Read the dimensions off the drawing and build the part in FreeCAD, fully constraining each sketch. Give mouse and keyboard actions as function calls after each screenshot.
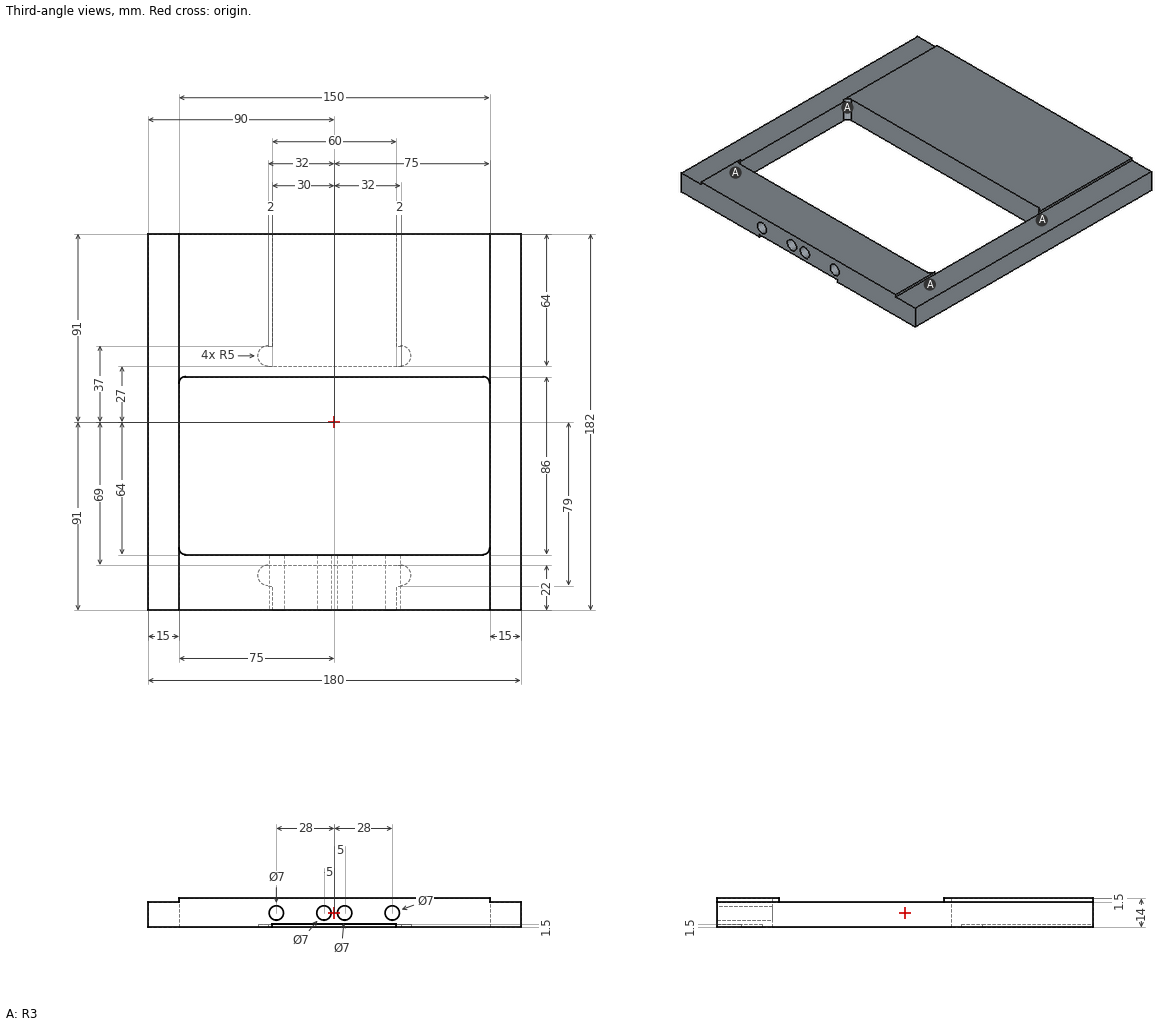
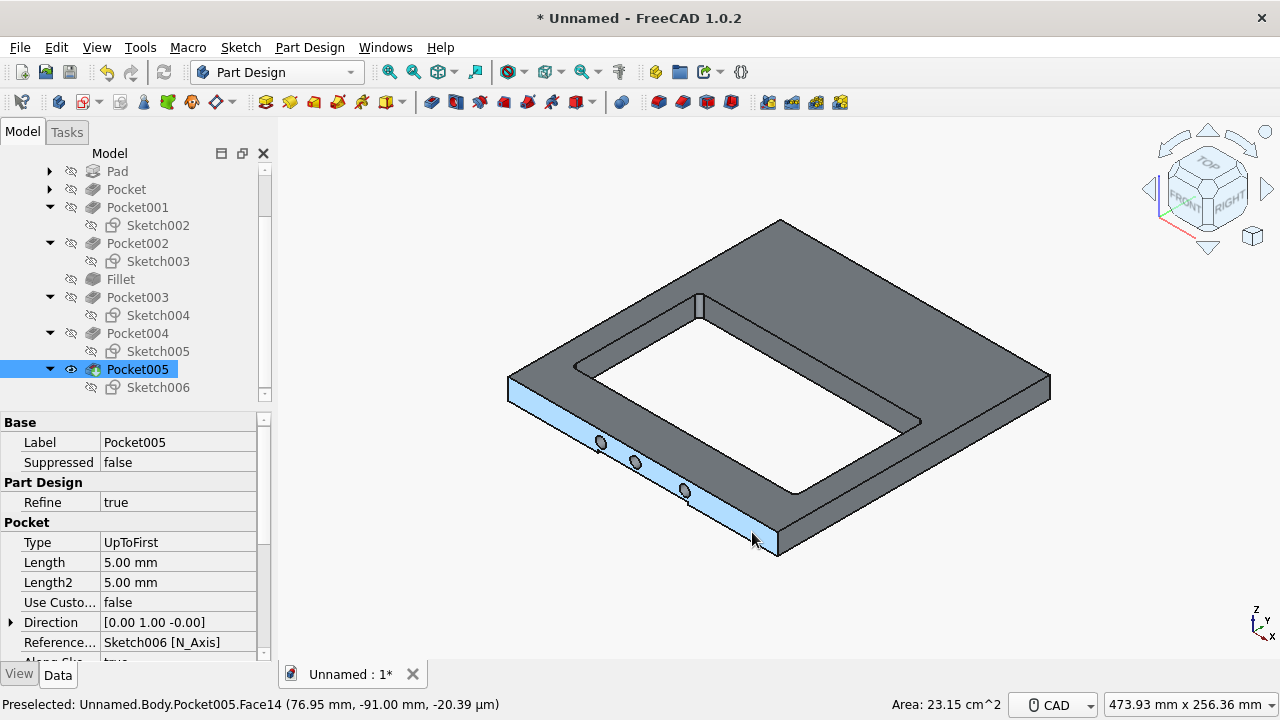
click(84, 102)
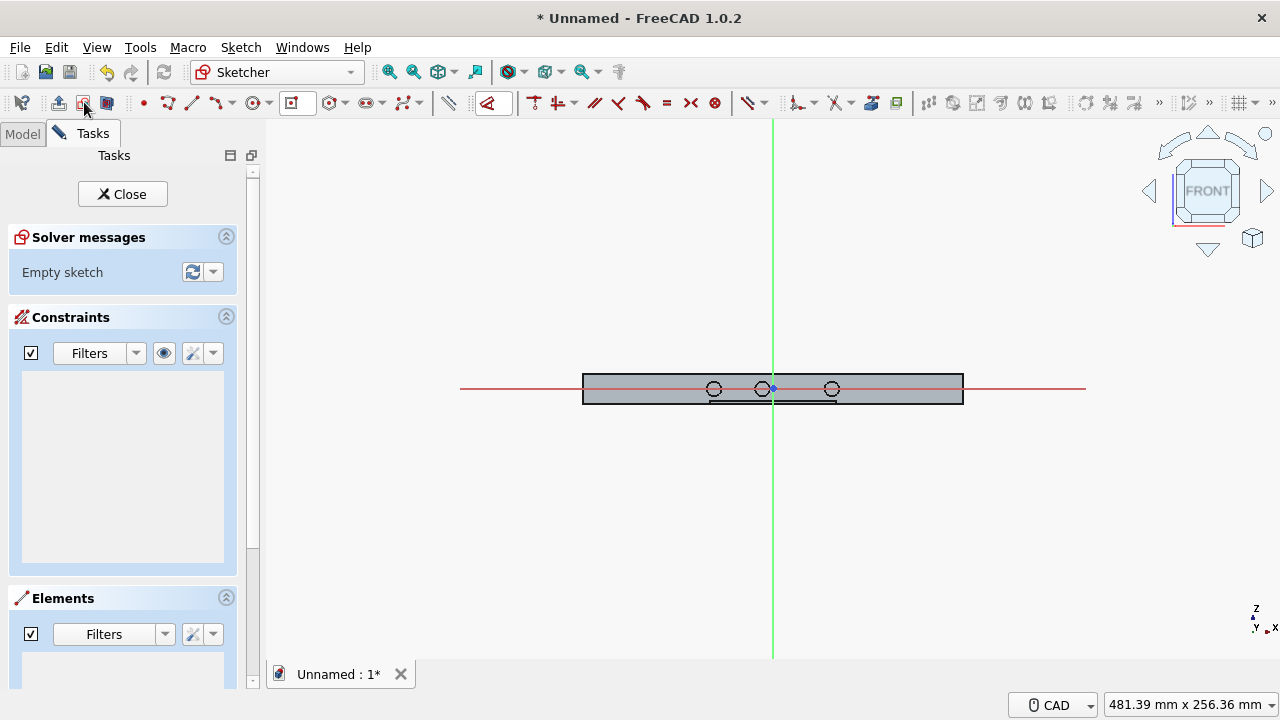
scroll(786, 389, up, 15)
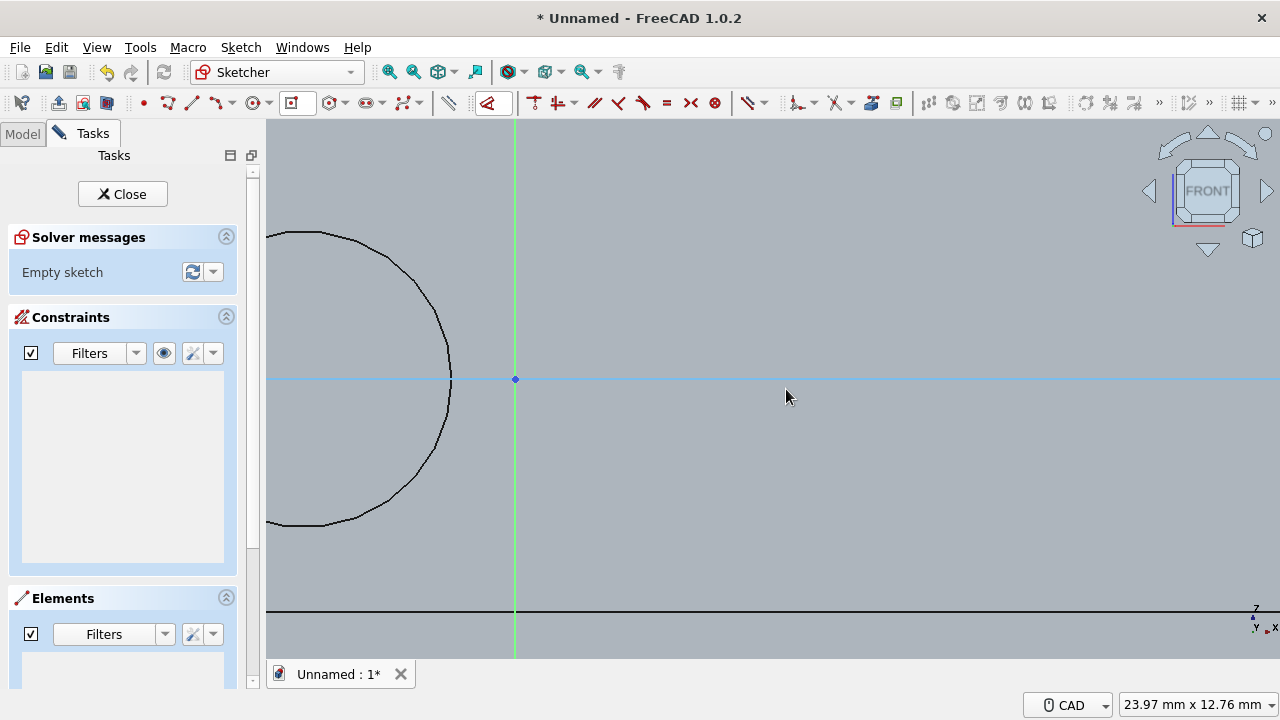
key(g)
key(c)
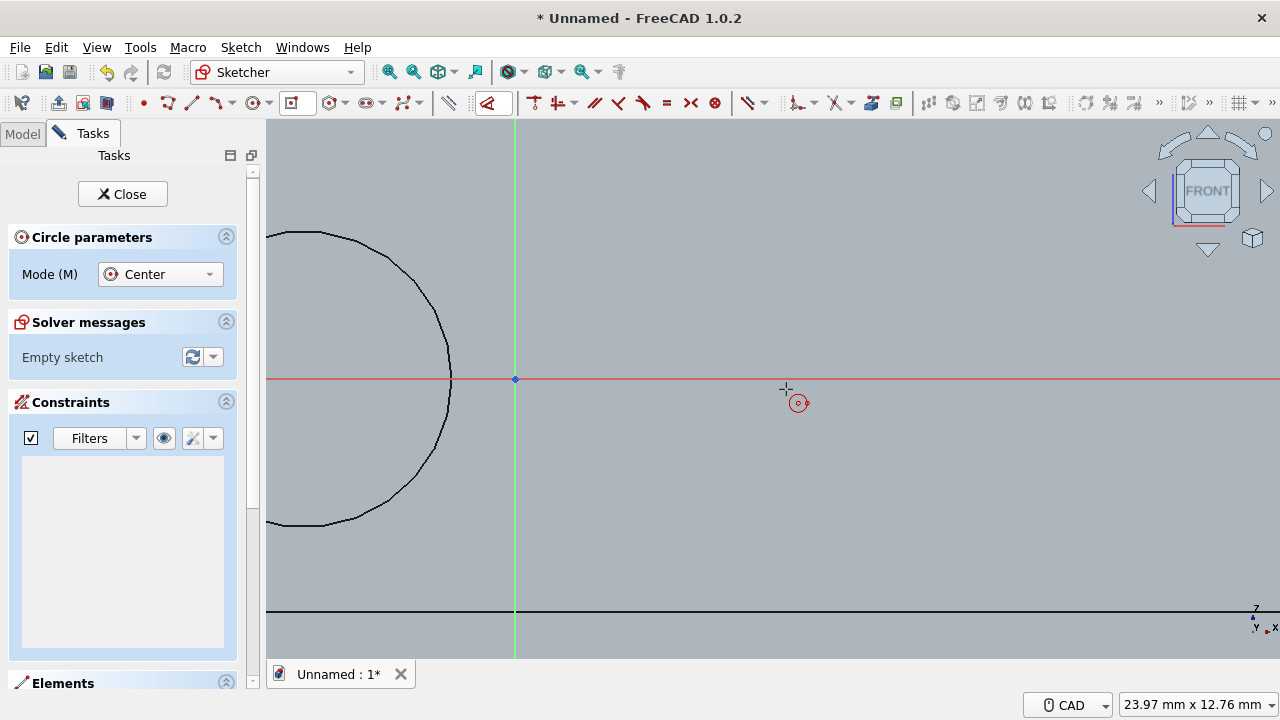
click(727, 379)
move(831, 275)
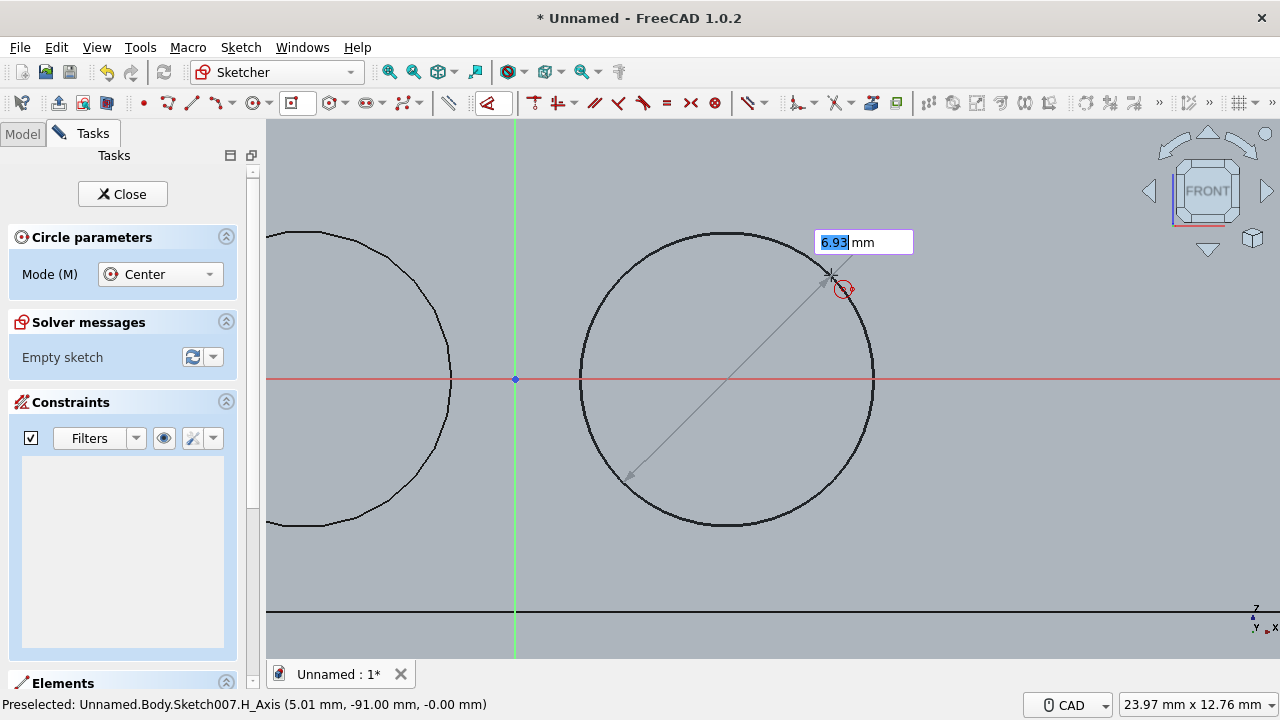
text(7)
key(Return)
key(Escape)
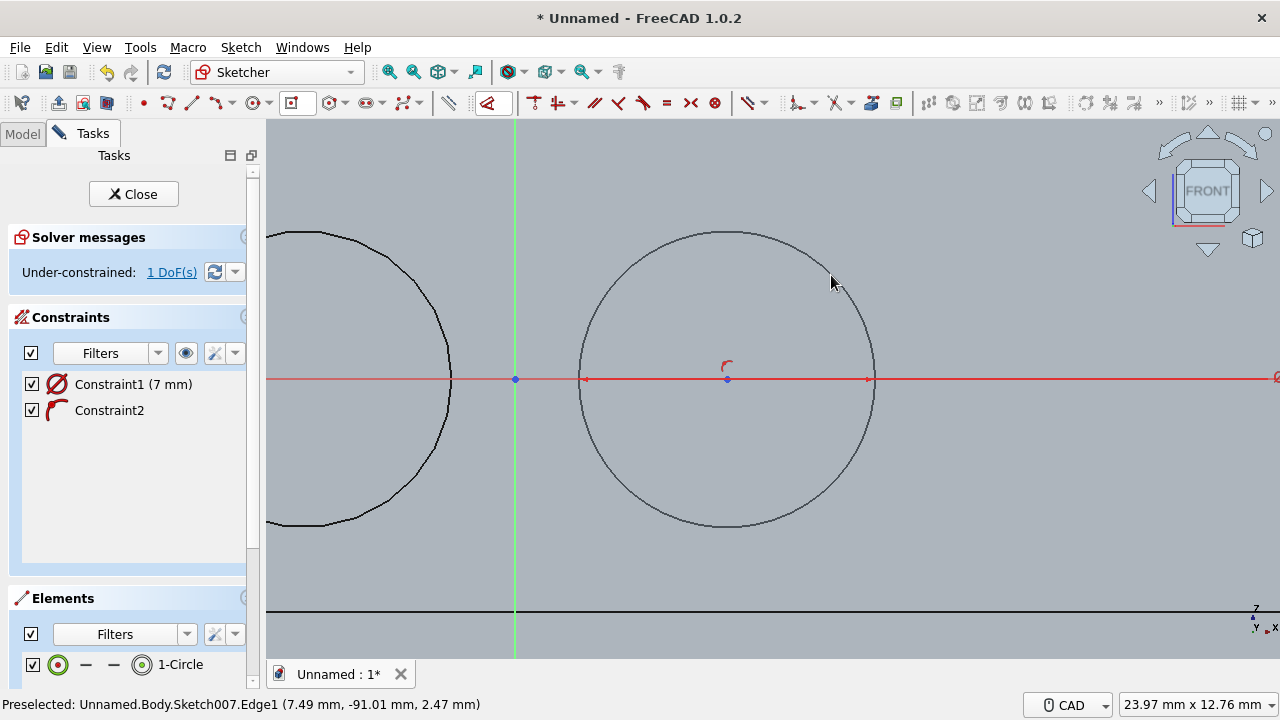
click(727, 379)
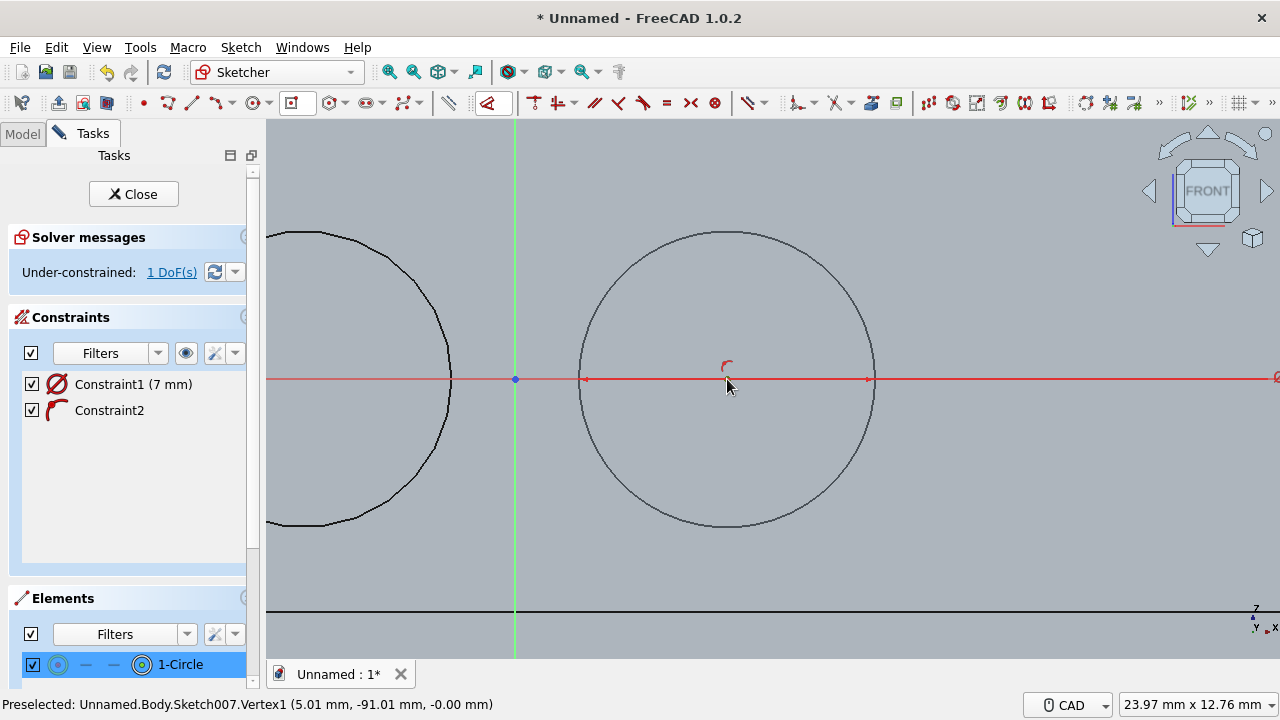
key(l)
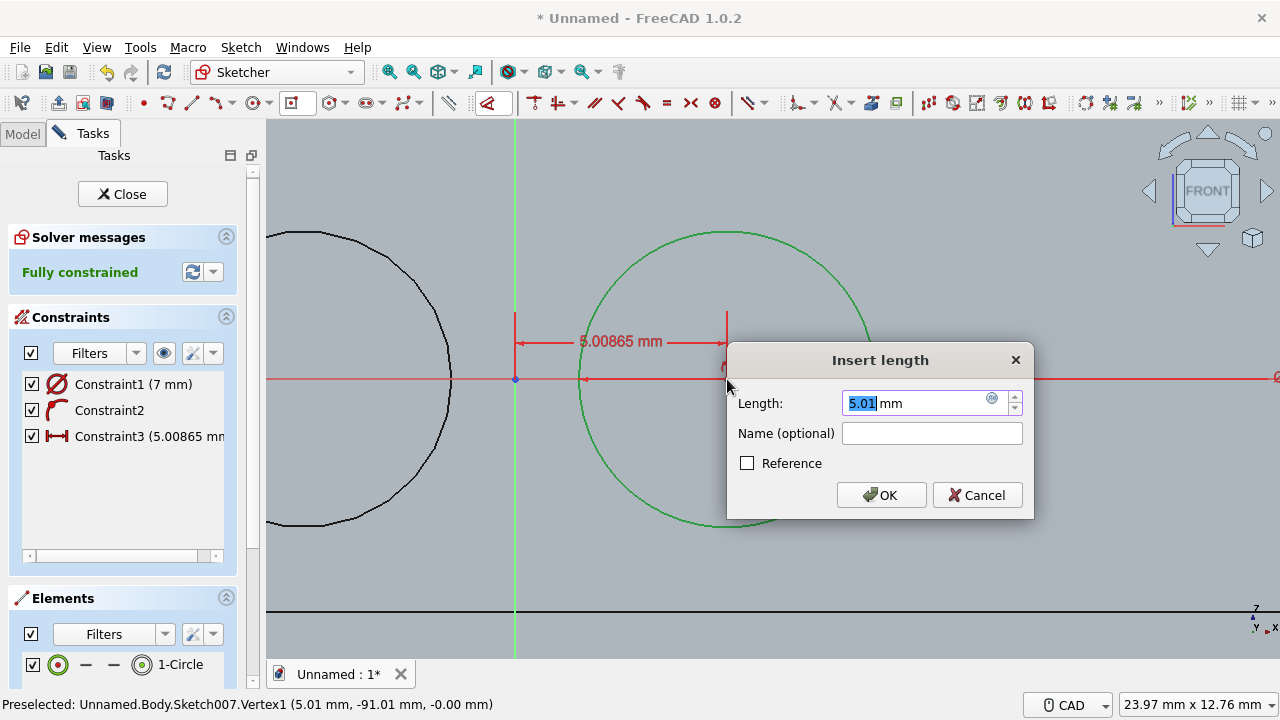
text(5)
key(Return)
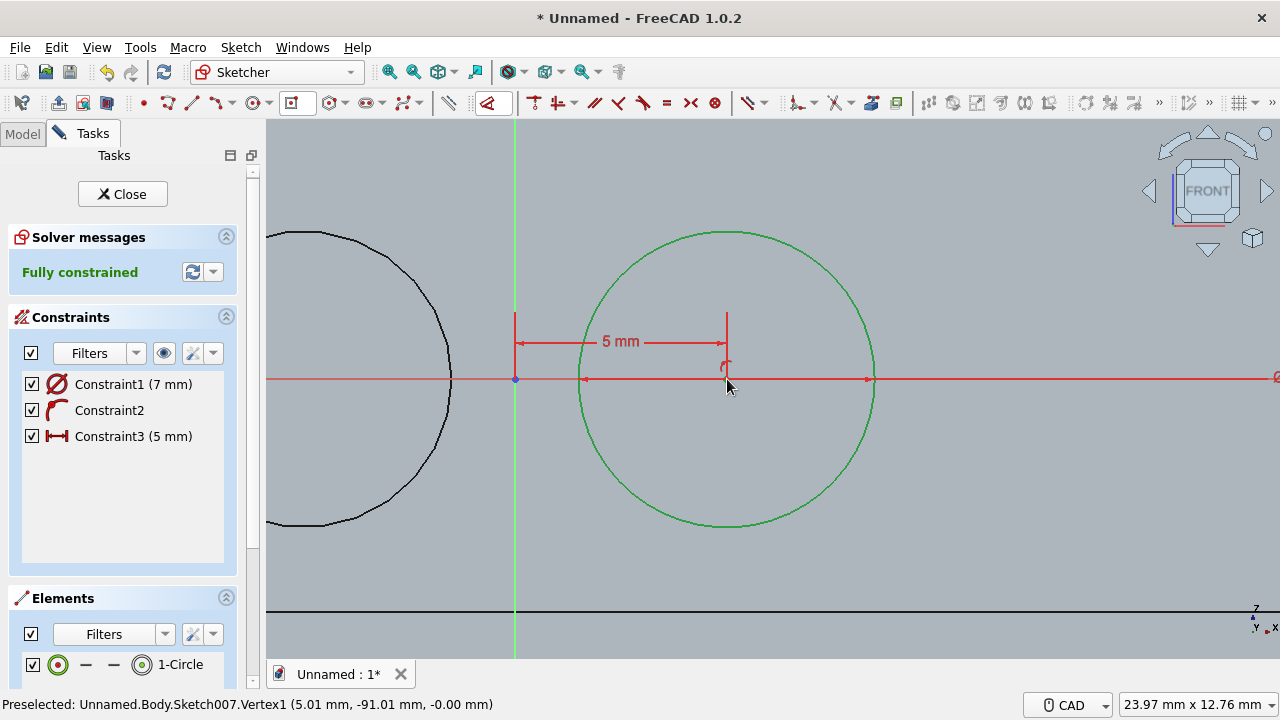
click(123, 194)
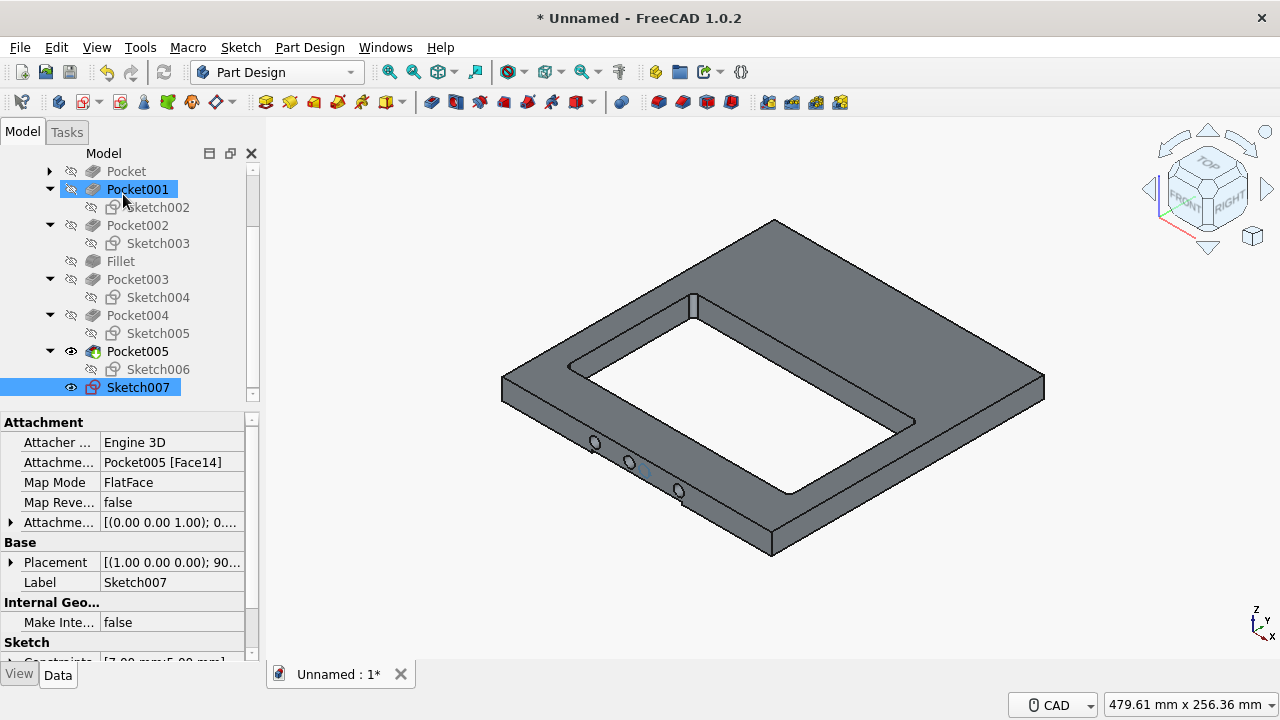
click(432, 102)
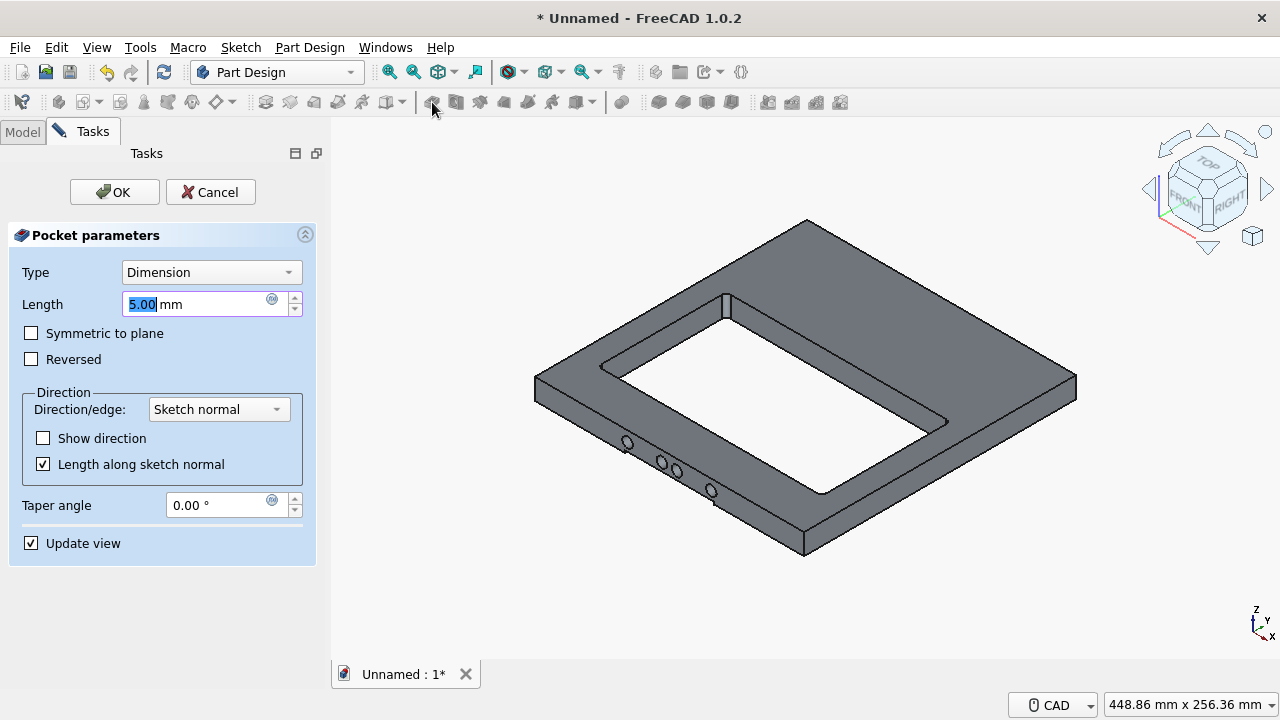
click(212, 272)